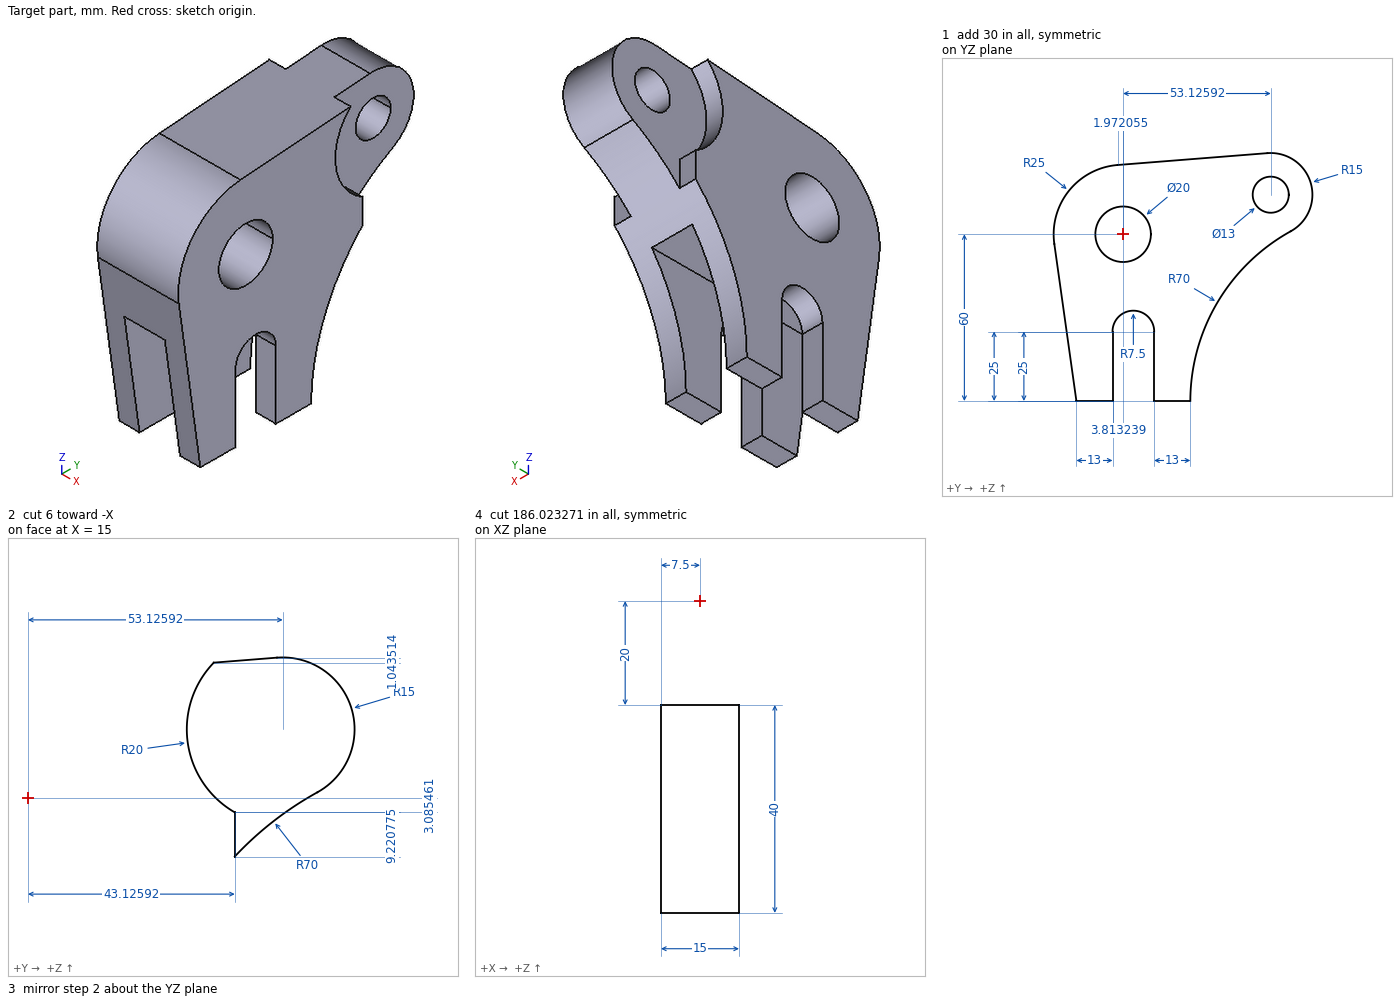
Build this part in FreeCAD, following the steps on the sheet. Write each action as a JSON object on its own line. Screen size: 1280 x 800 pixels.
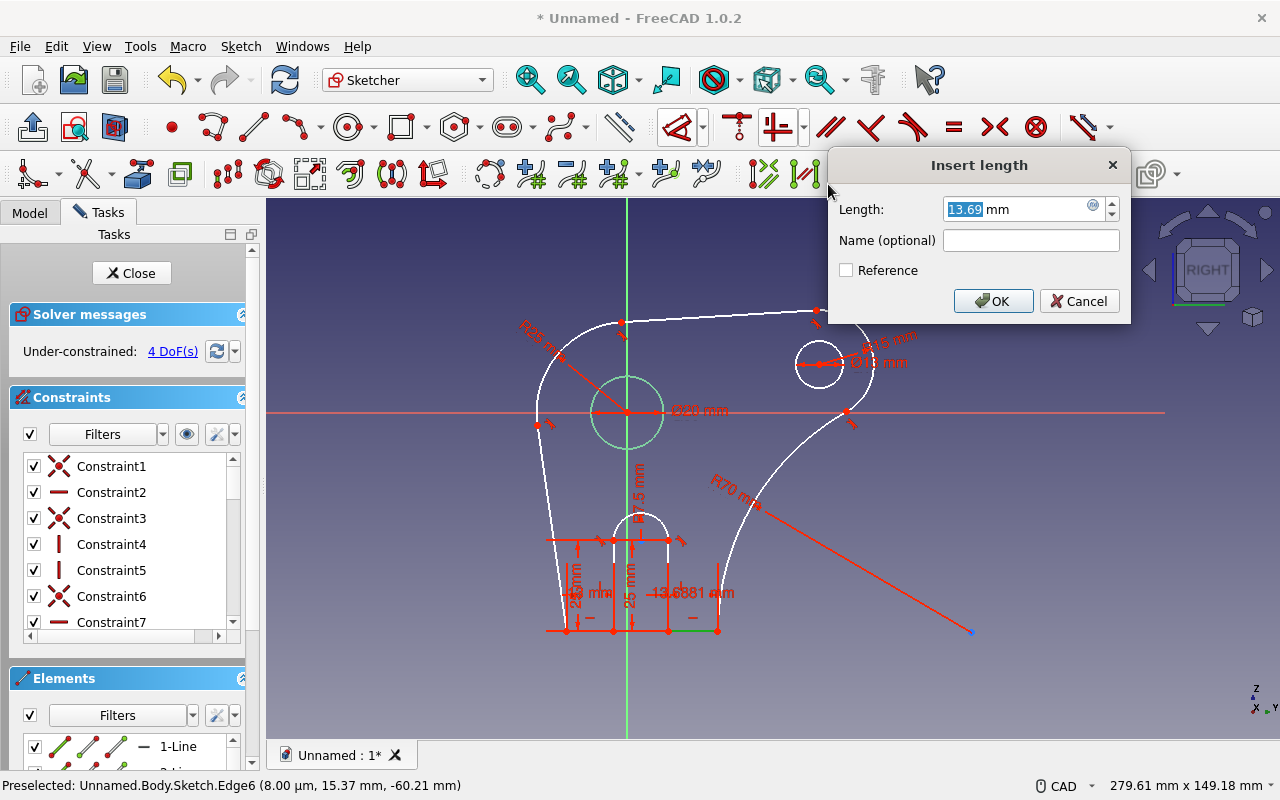
{"action": "type", "text": "13"}
{"action": "key", "text": "Return"}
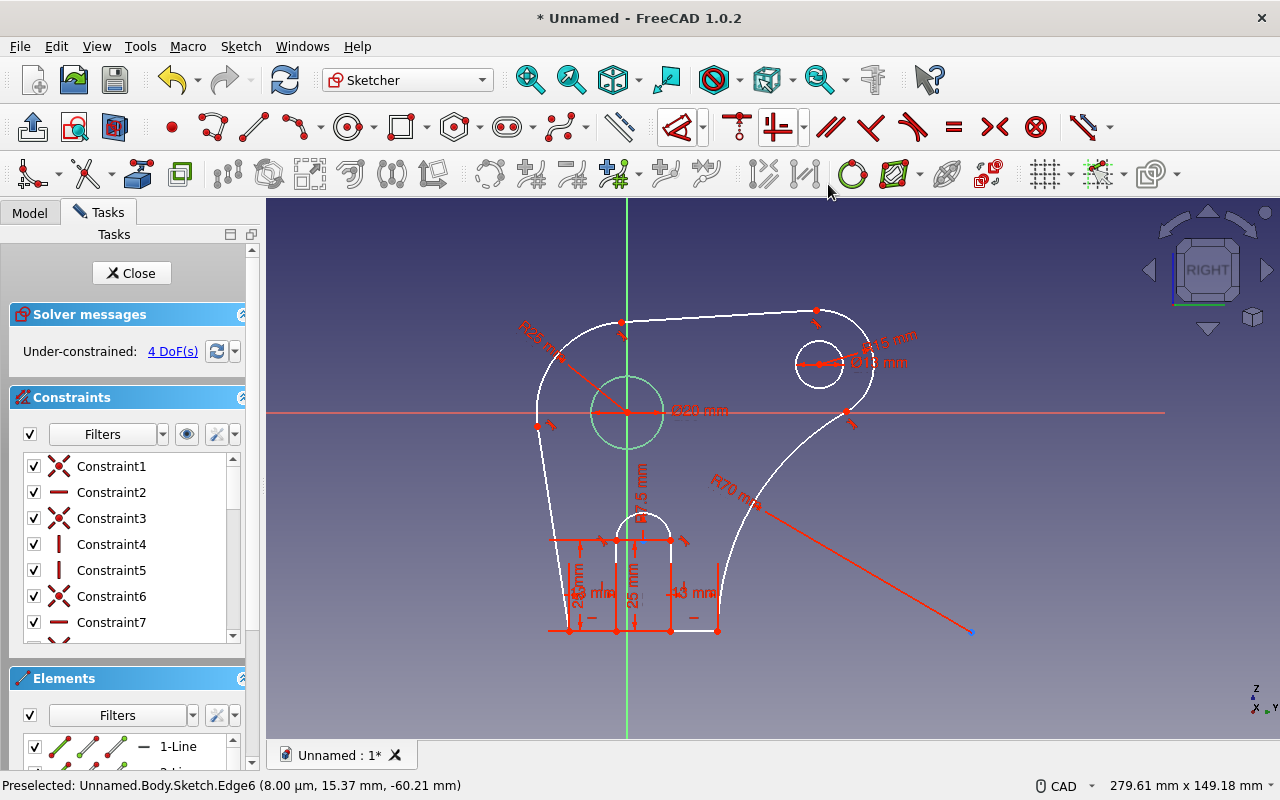
{"action": "left_click", "coordinate": [569, 631]}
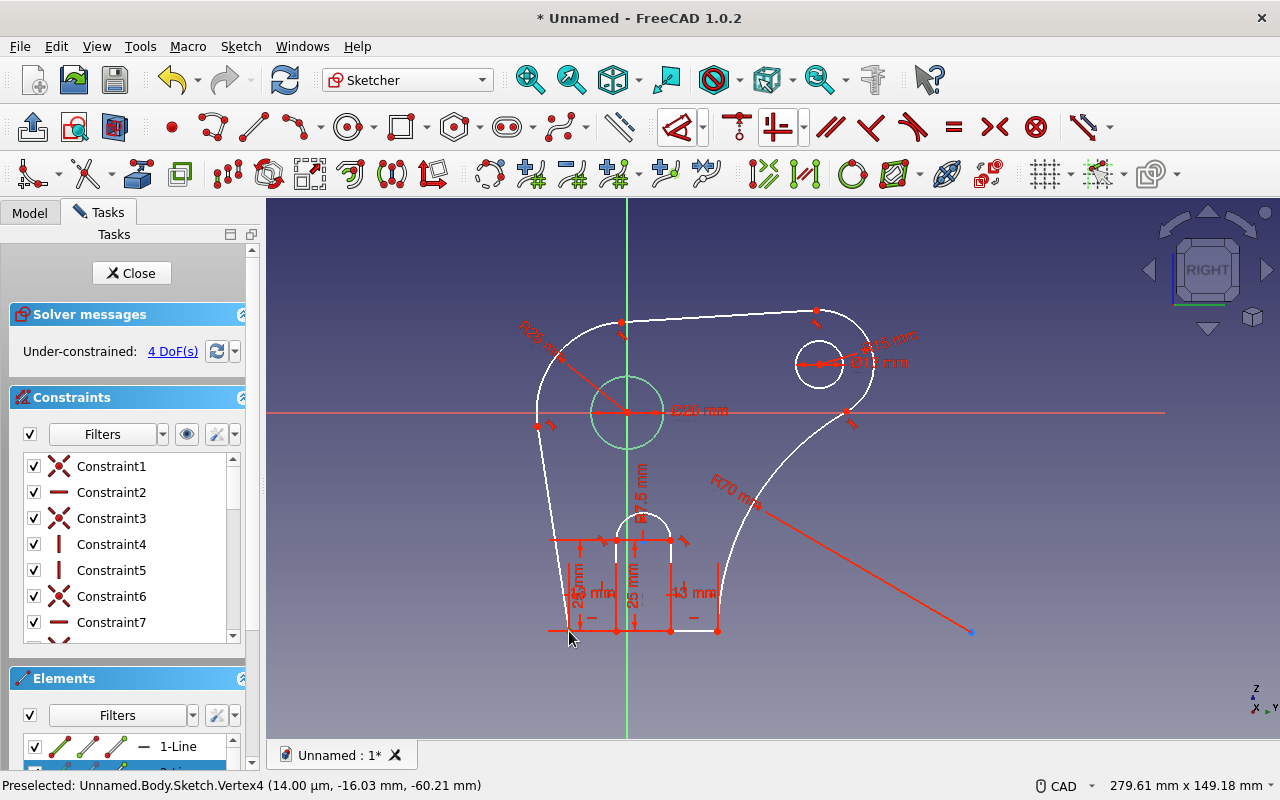
{"action": "key", "text": "i"}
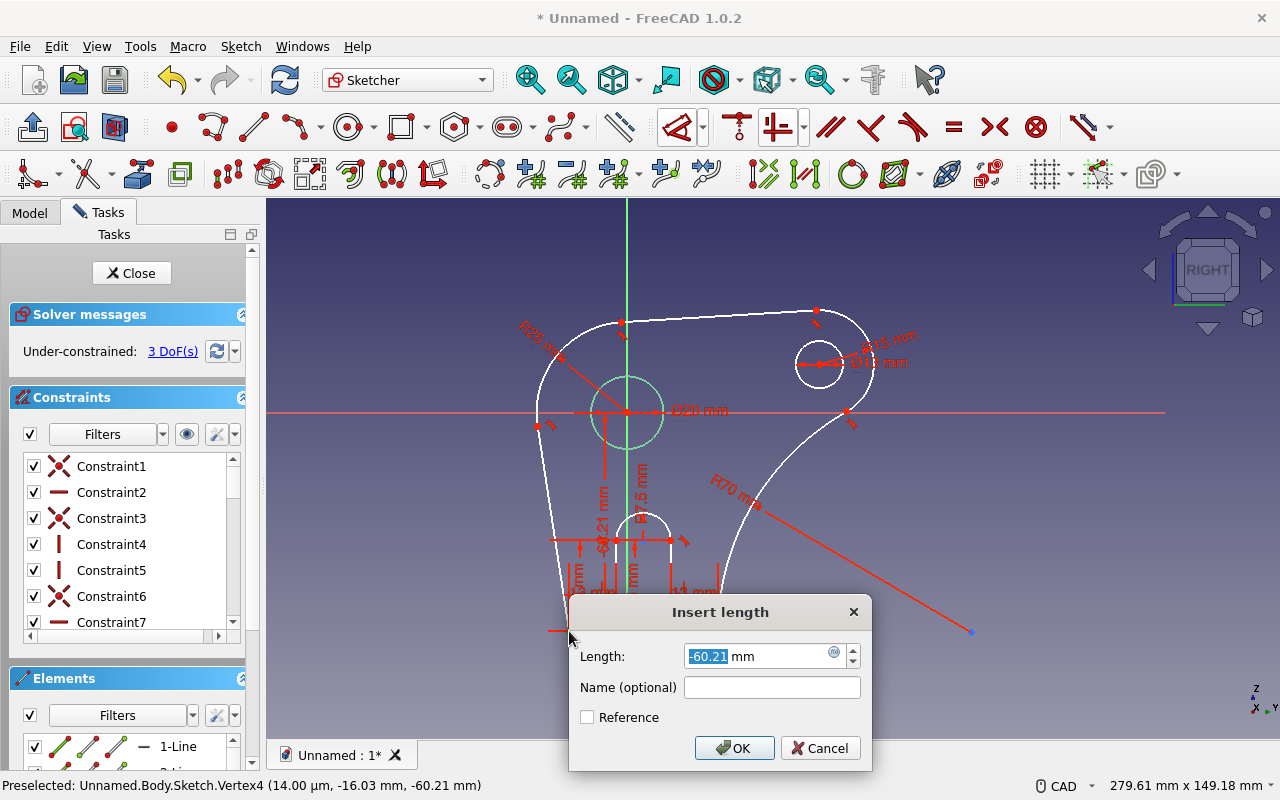
{"action": "type", "text": "-60"}
{"action": "key", "text": "Return"}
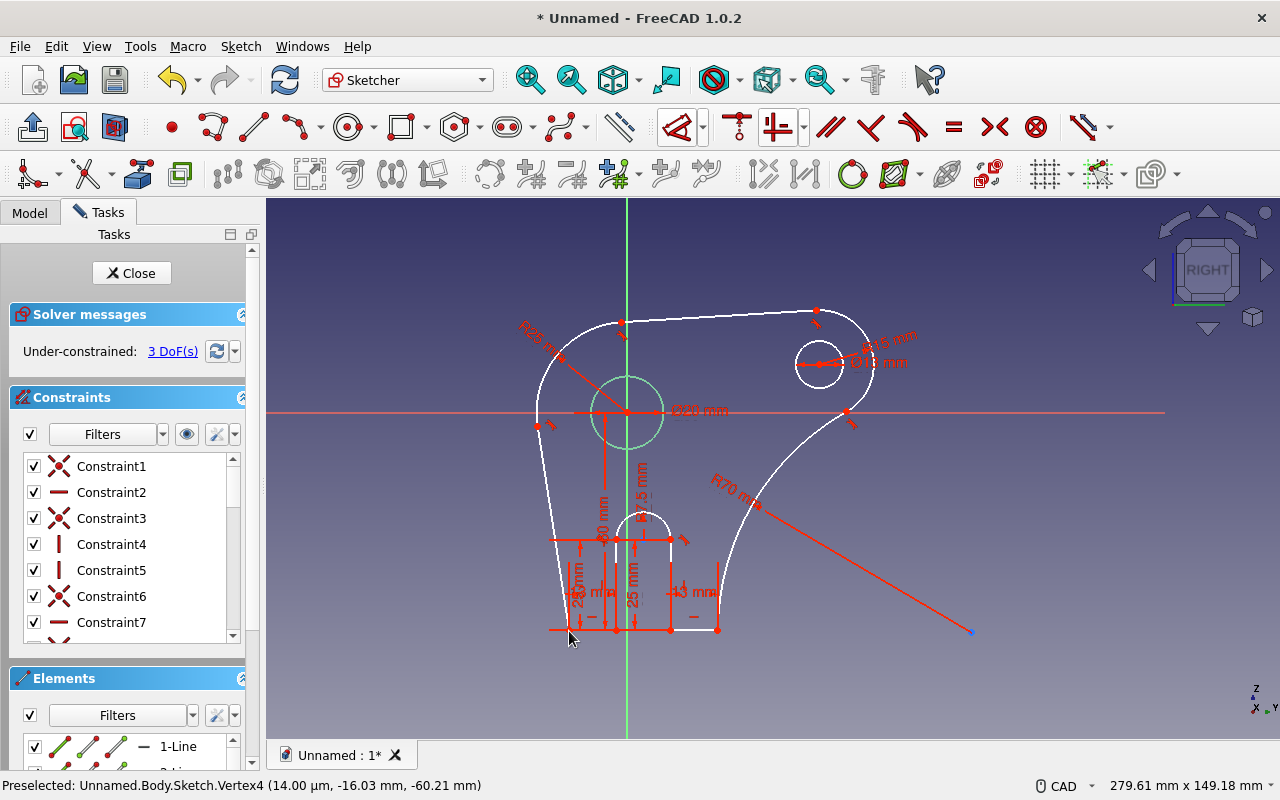
{"action": "left_click", "coordinate": [819, 365]}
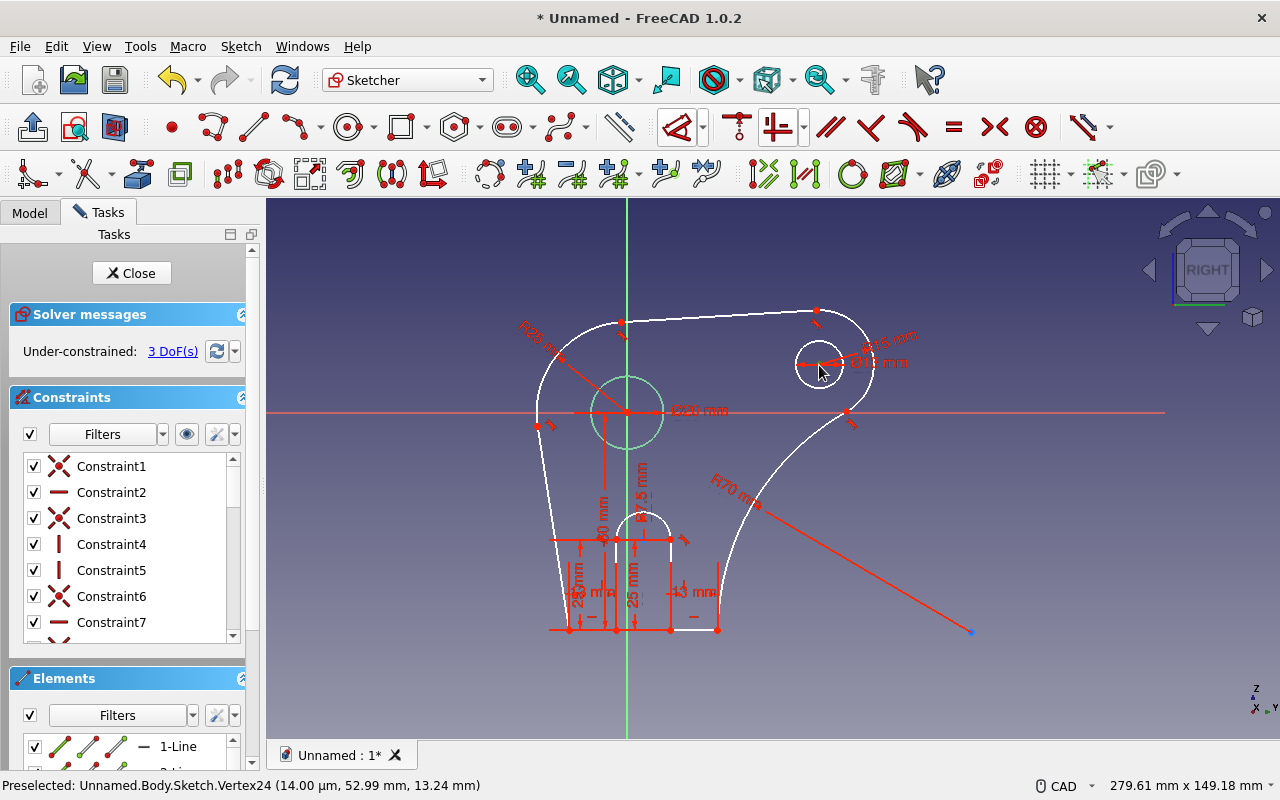
{"action": "key", "text": "l"}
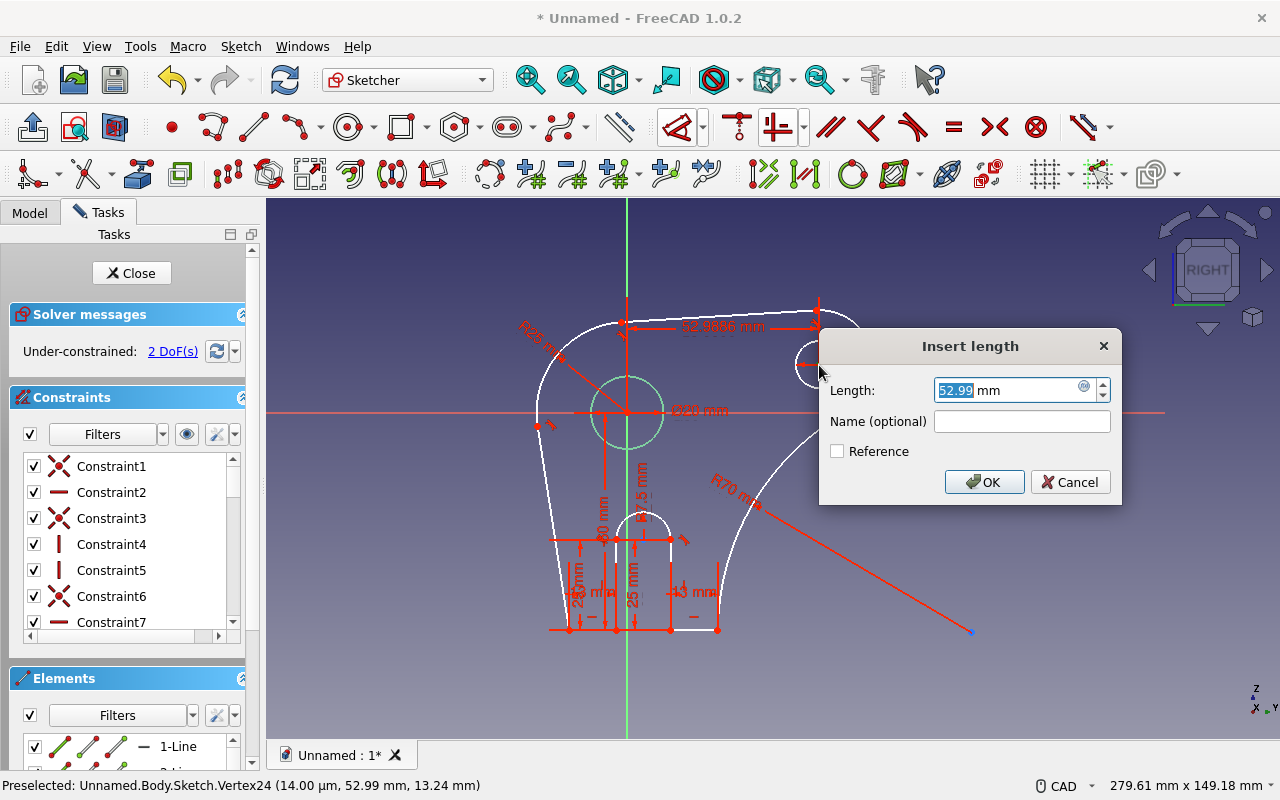
{"action": "type", "text": "53.12592"}
{"action": "key", "text": "Return"}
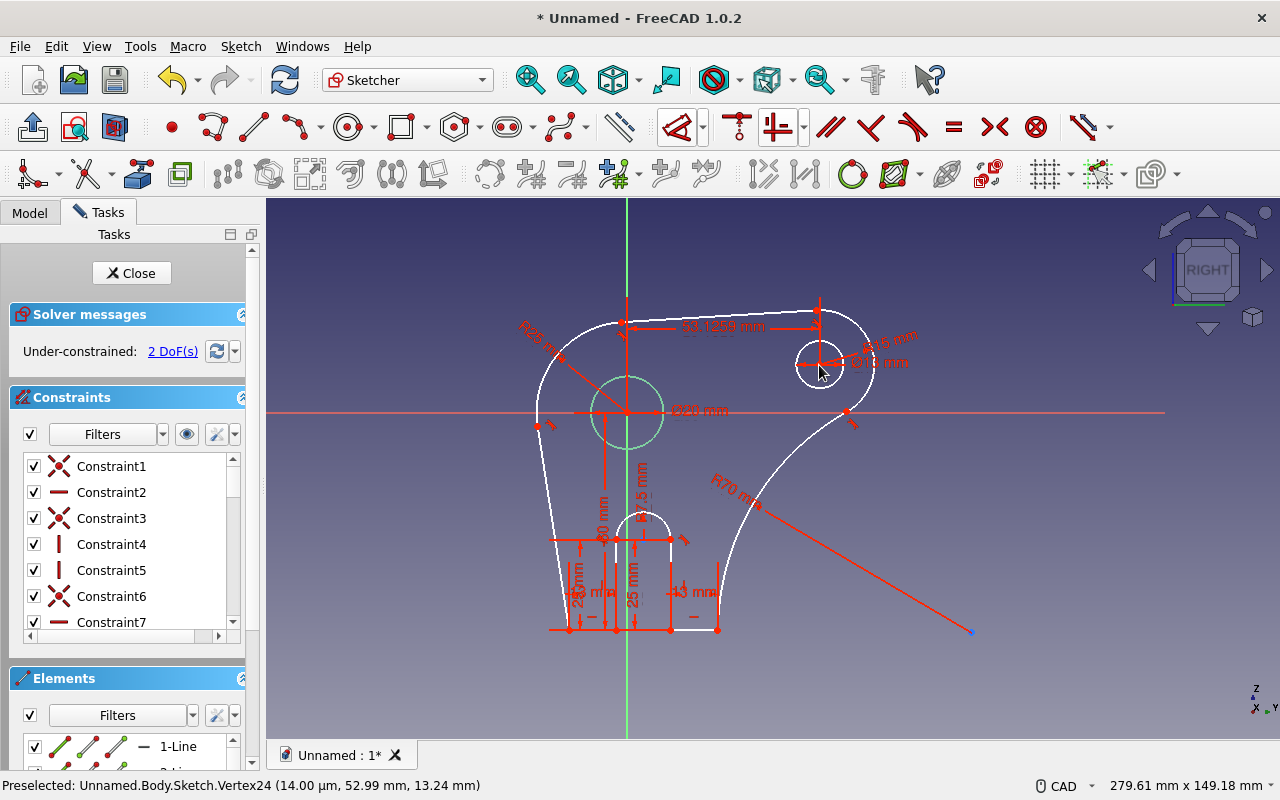
{"action": "scroll", "coordinate": [622, 322], "scroll_direction": "up", "scroll_amount": 9}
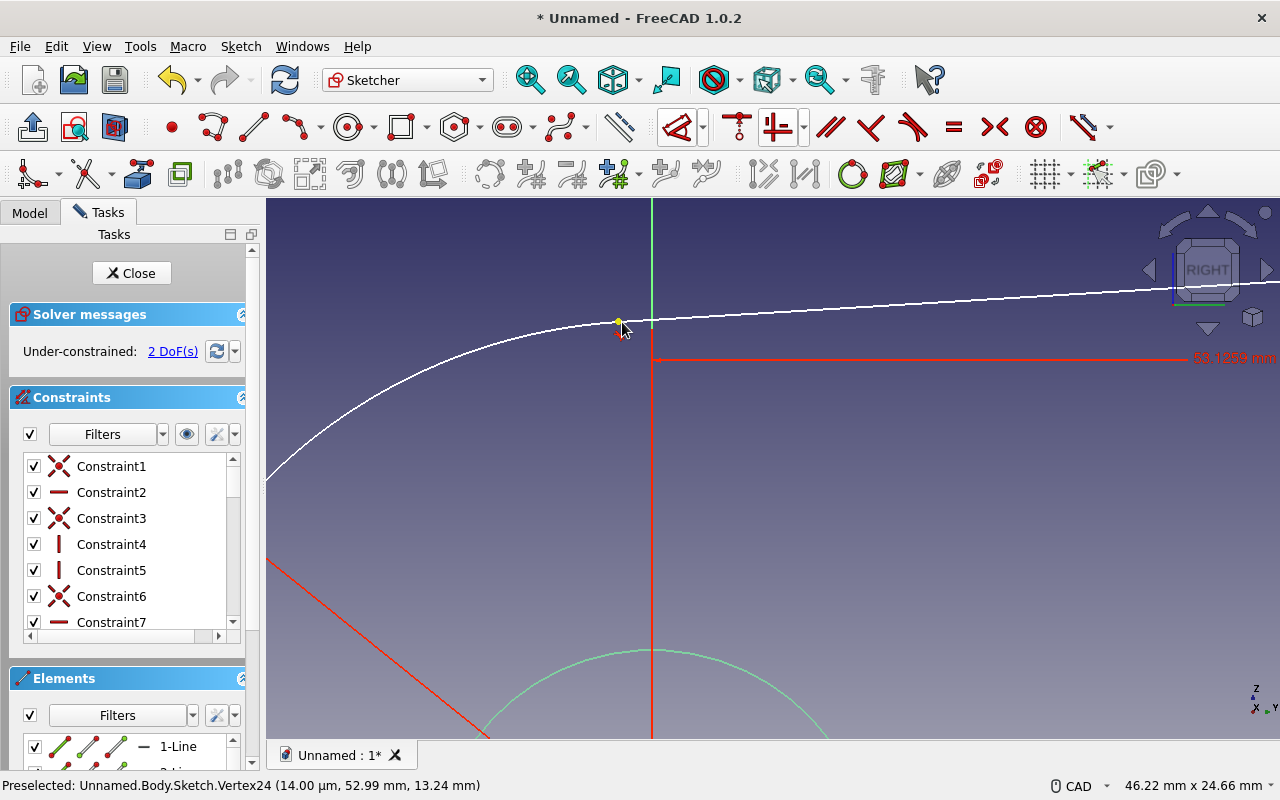
{"action": "left_click", "coordinate": [619, 322]}